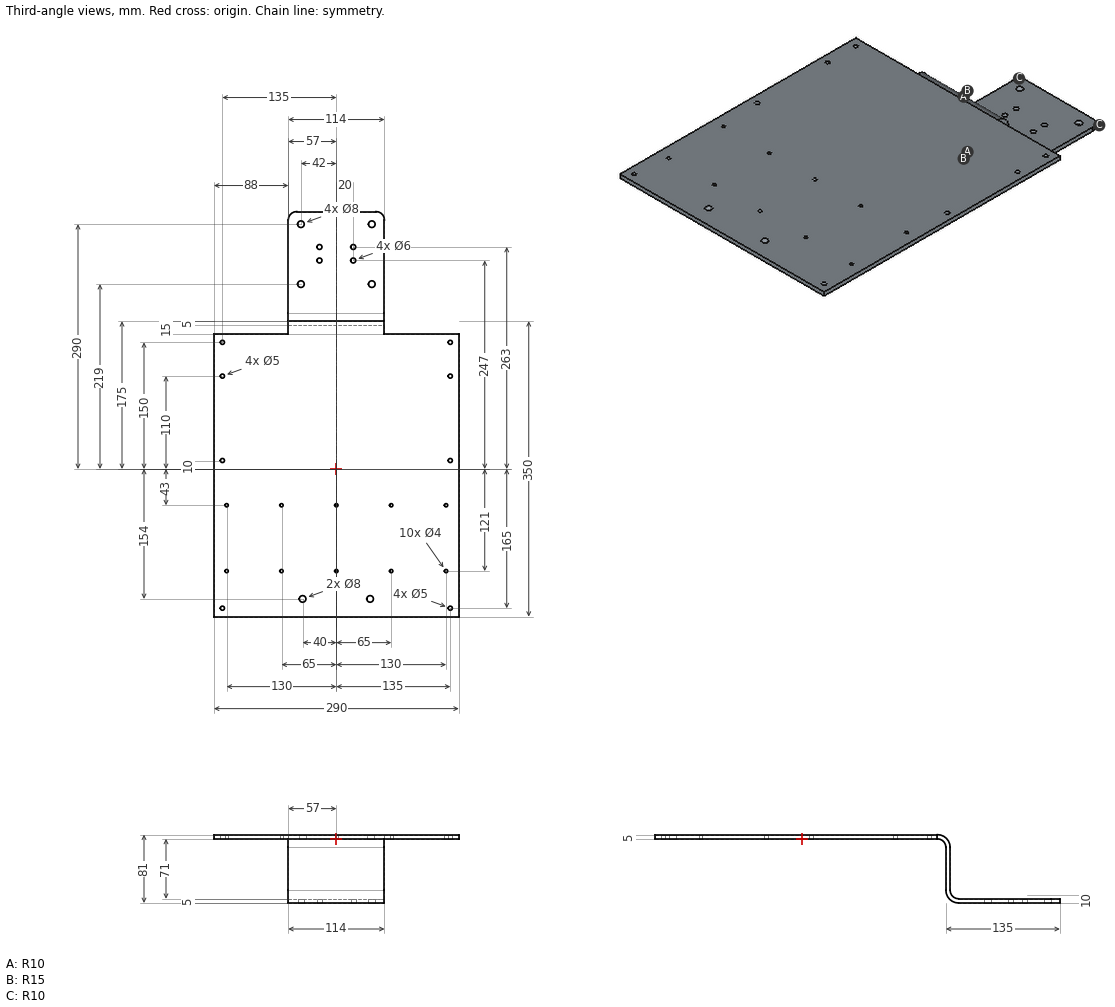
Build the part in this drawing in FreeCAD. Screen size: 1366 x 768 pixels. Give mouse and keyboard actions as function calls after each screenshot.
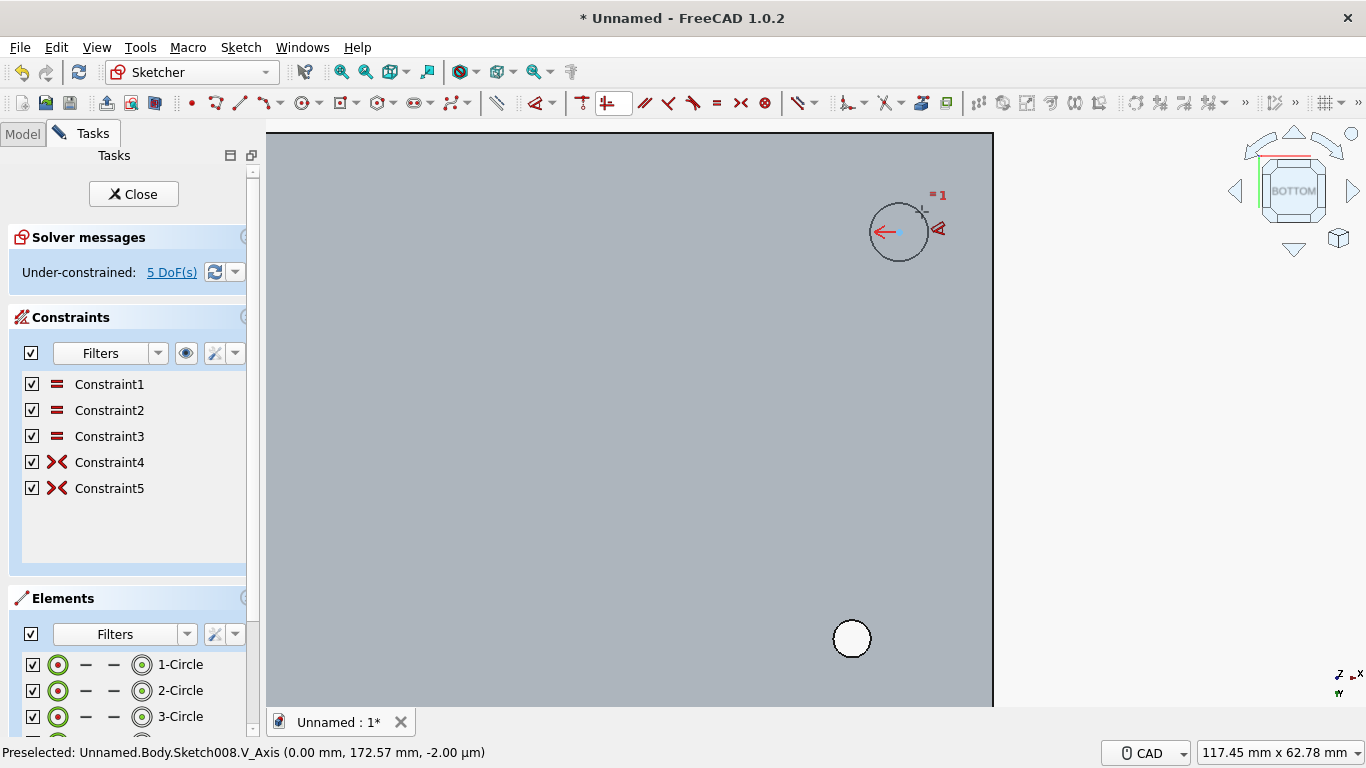
click(920, 212)
click(943, 190)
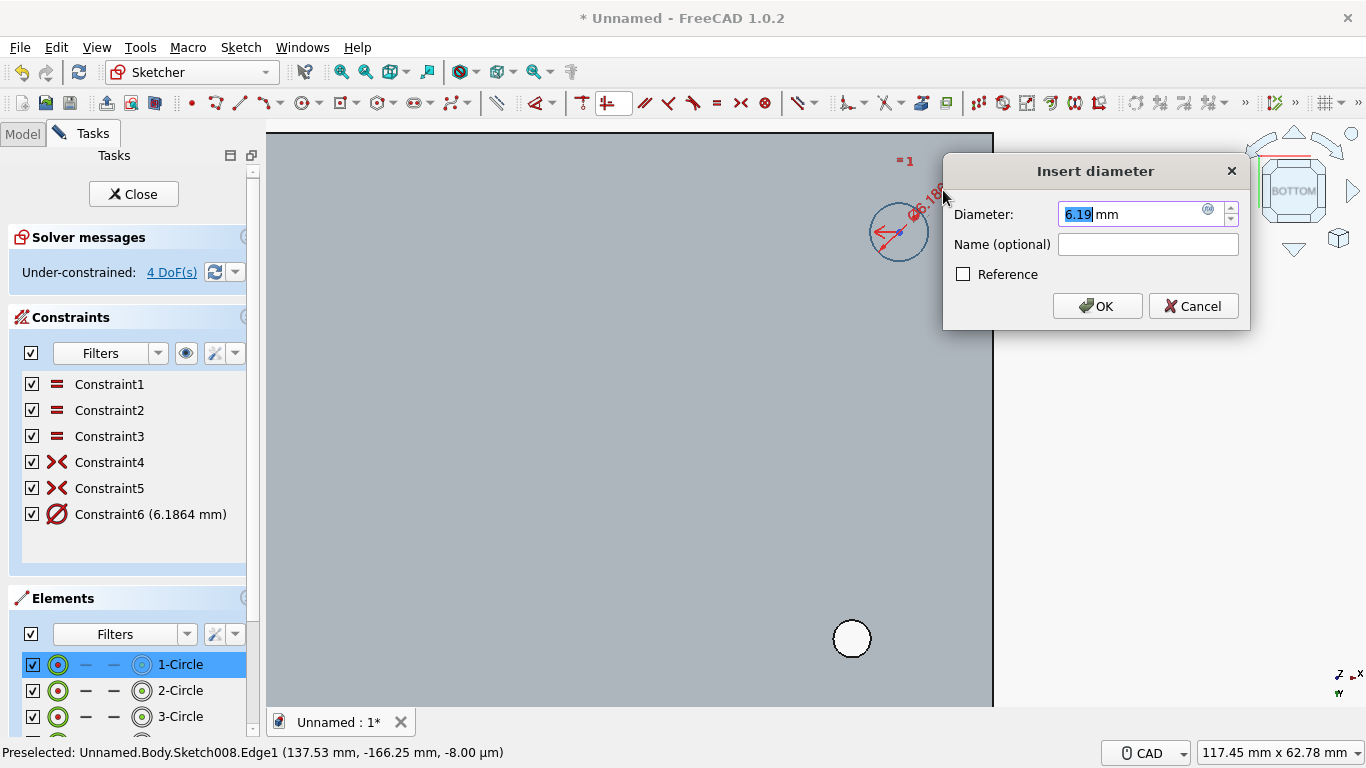
text(5)
key(Return)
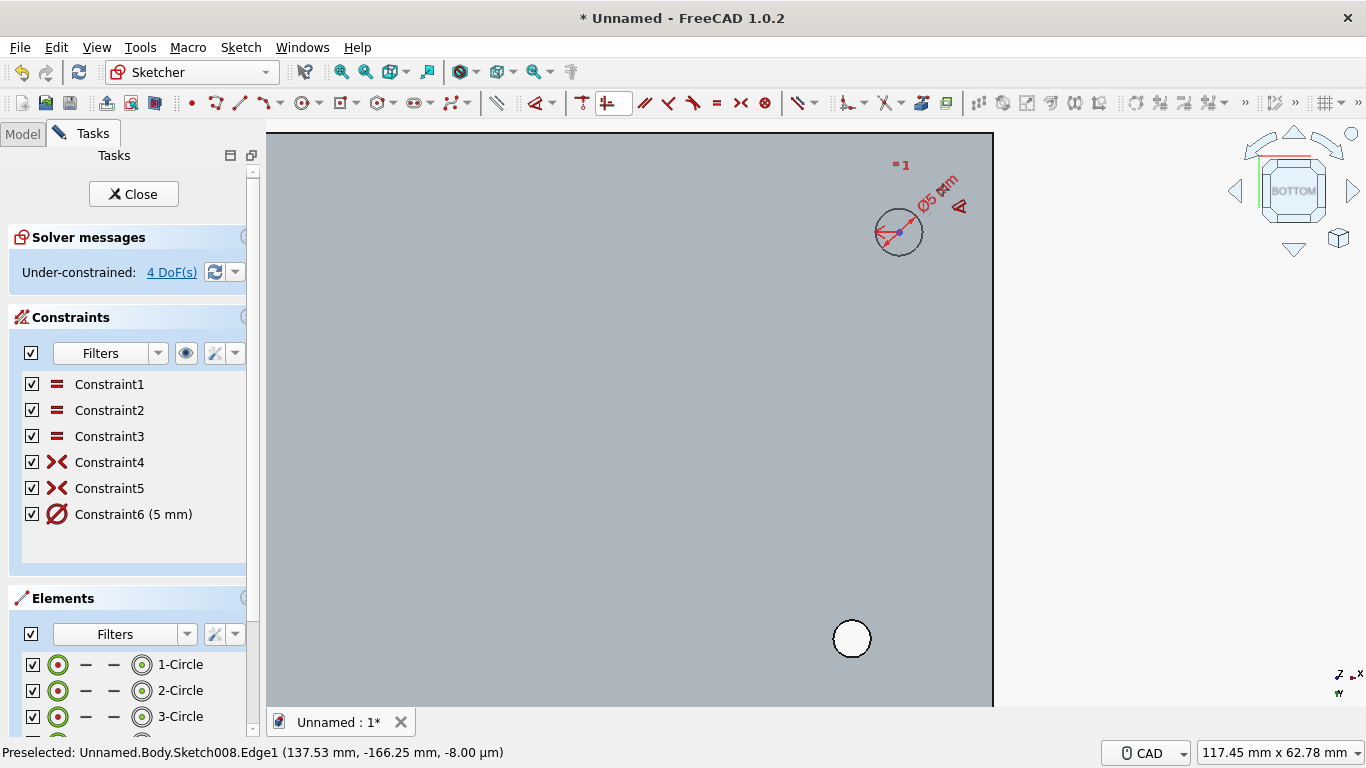
scroll(922, 211, down, 10)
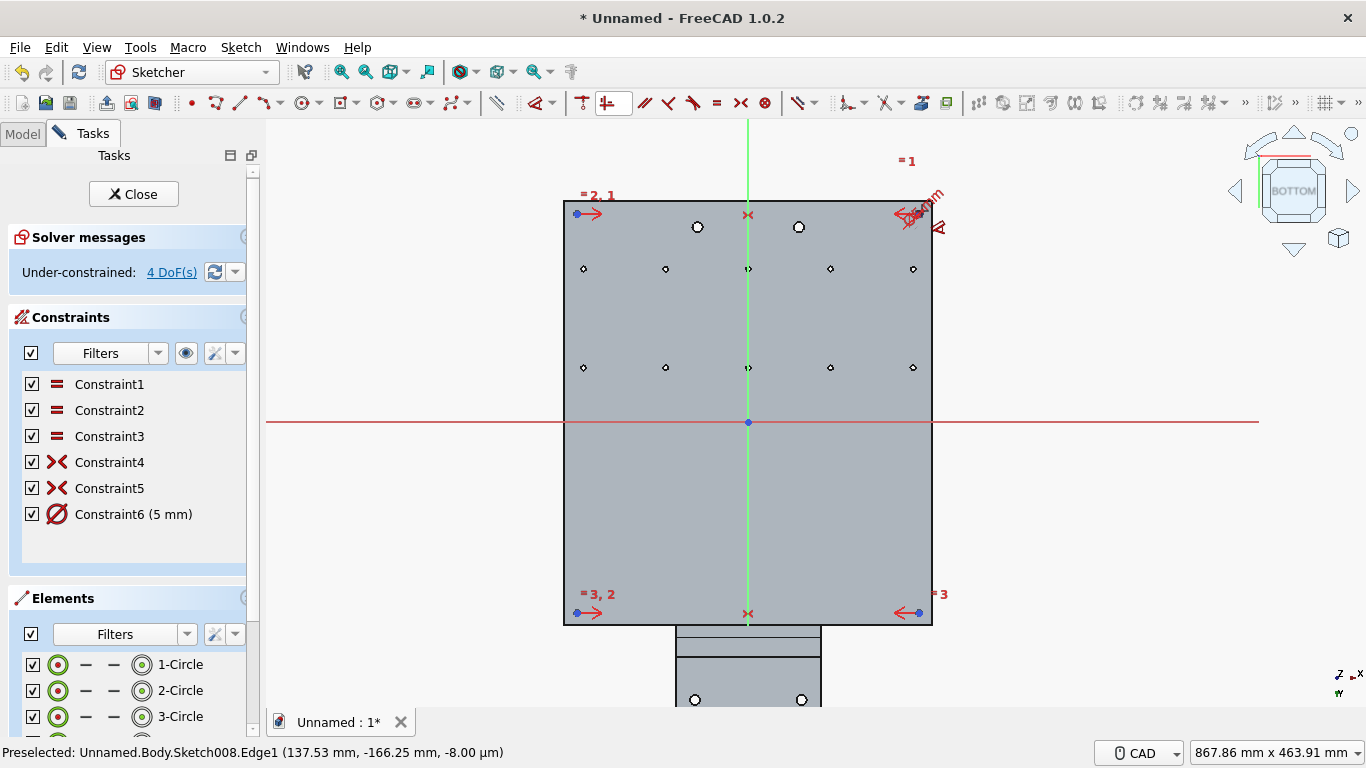
click(919, 214)
click(834, 180)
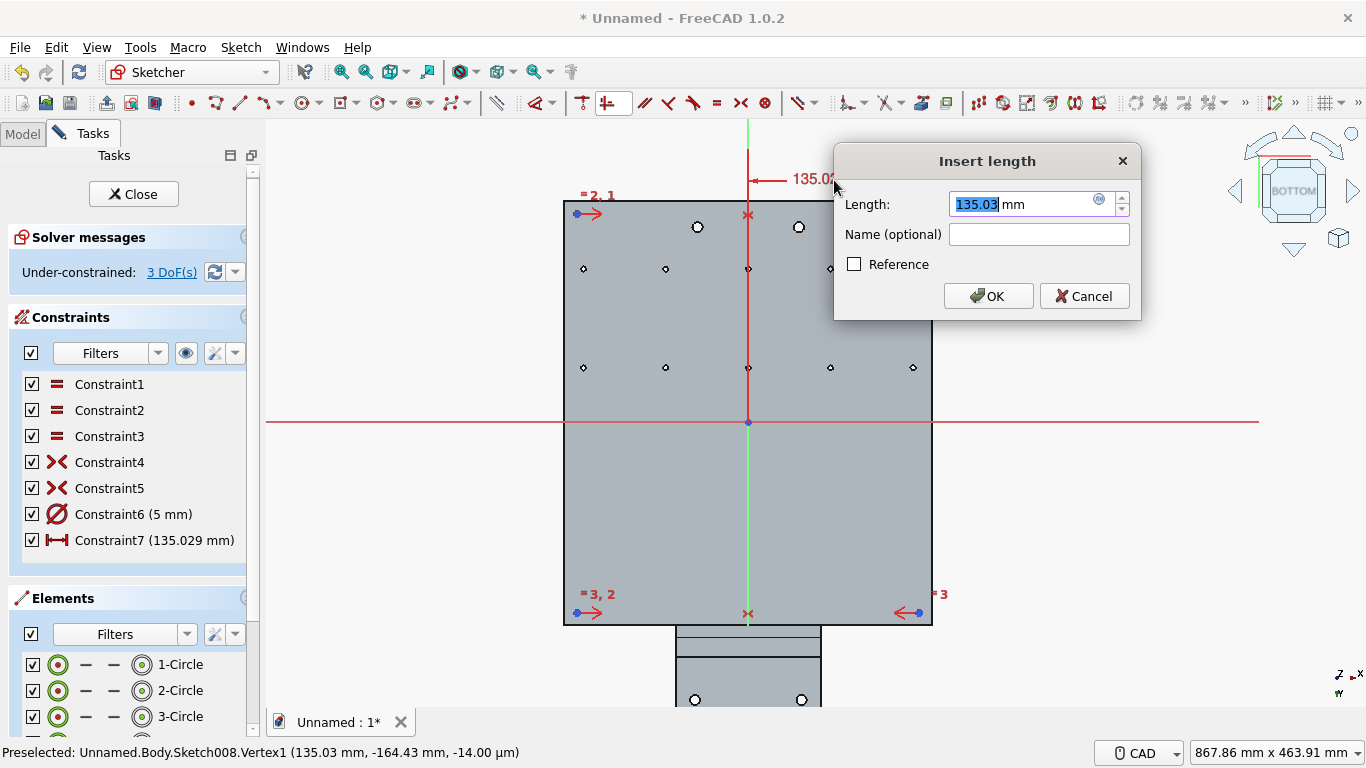
text(135)
key(Return)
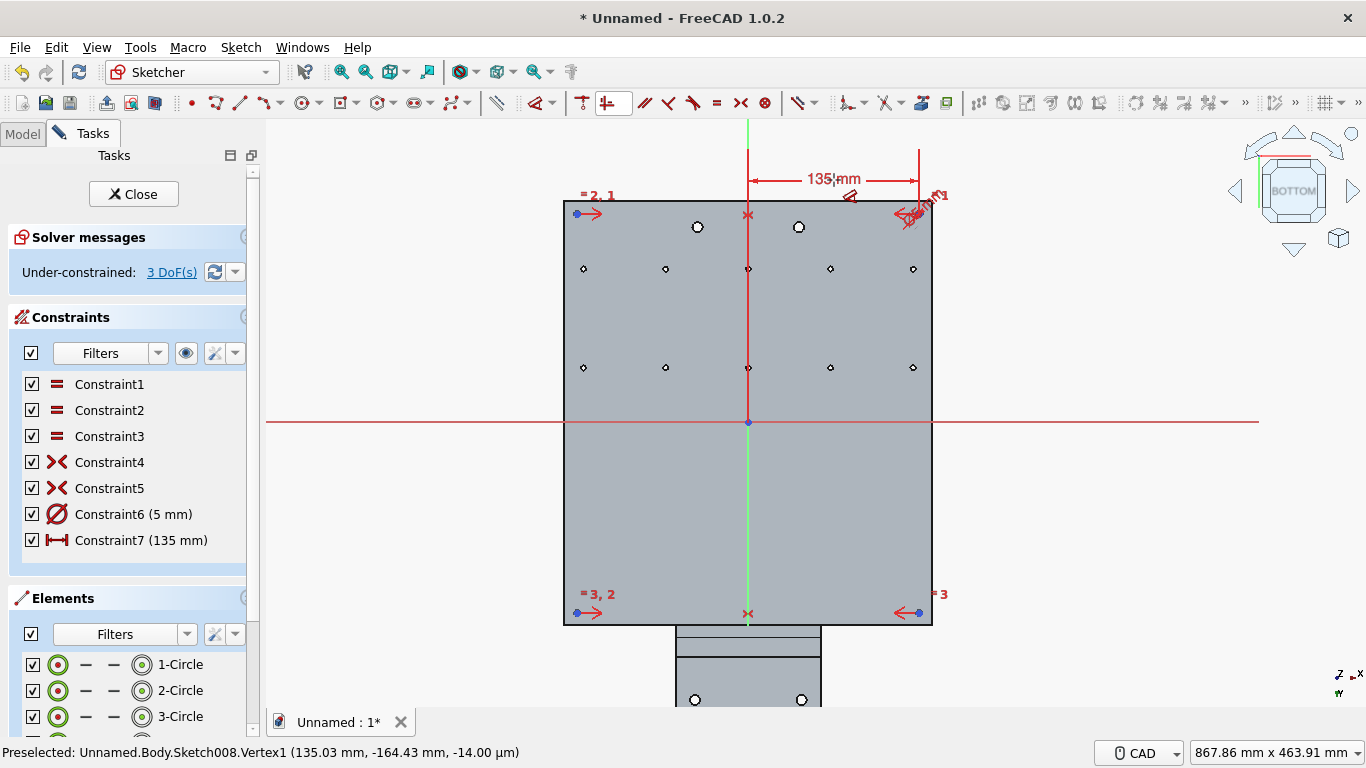
click(919, 214)
click(953, 318)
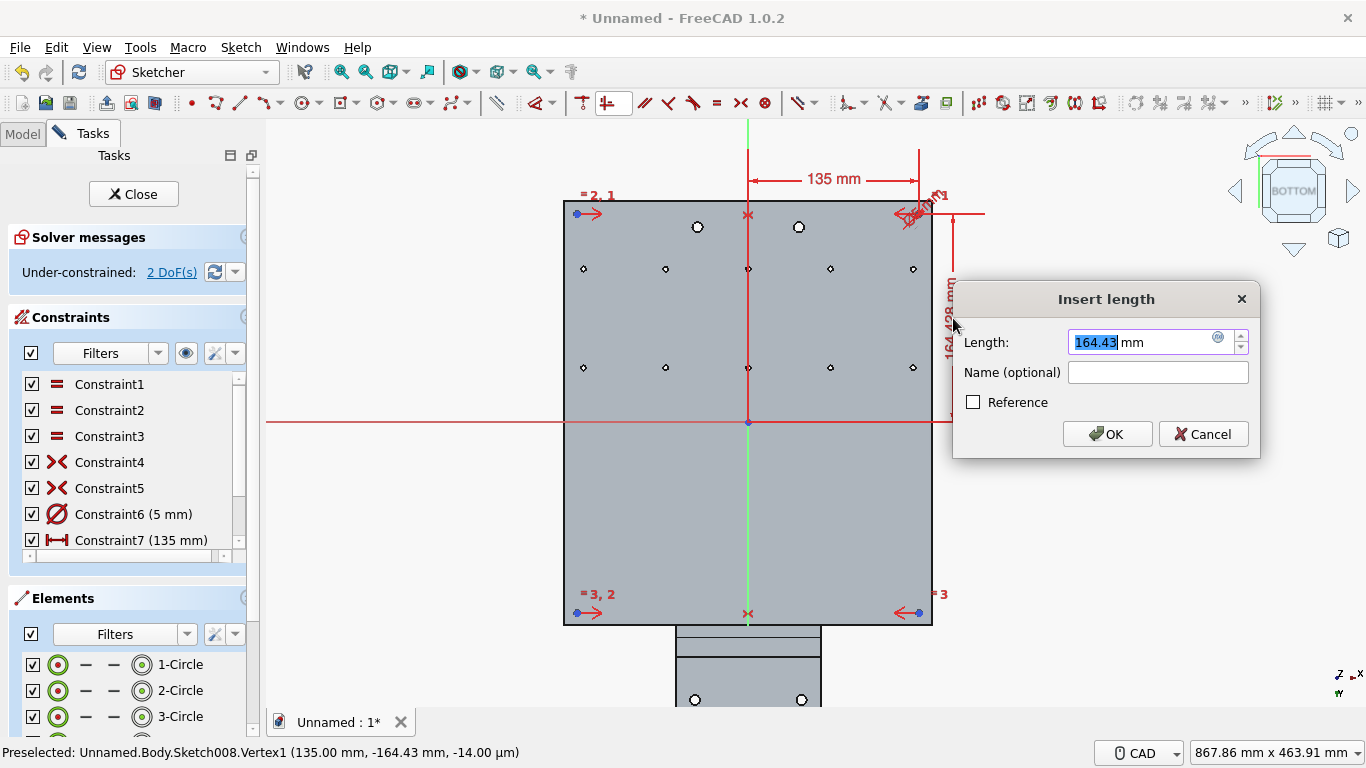
text(165)
key(Return)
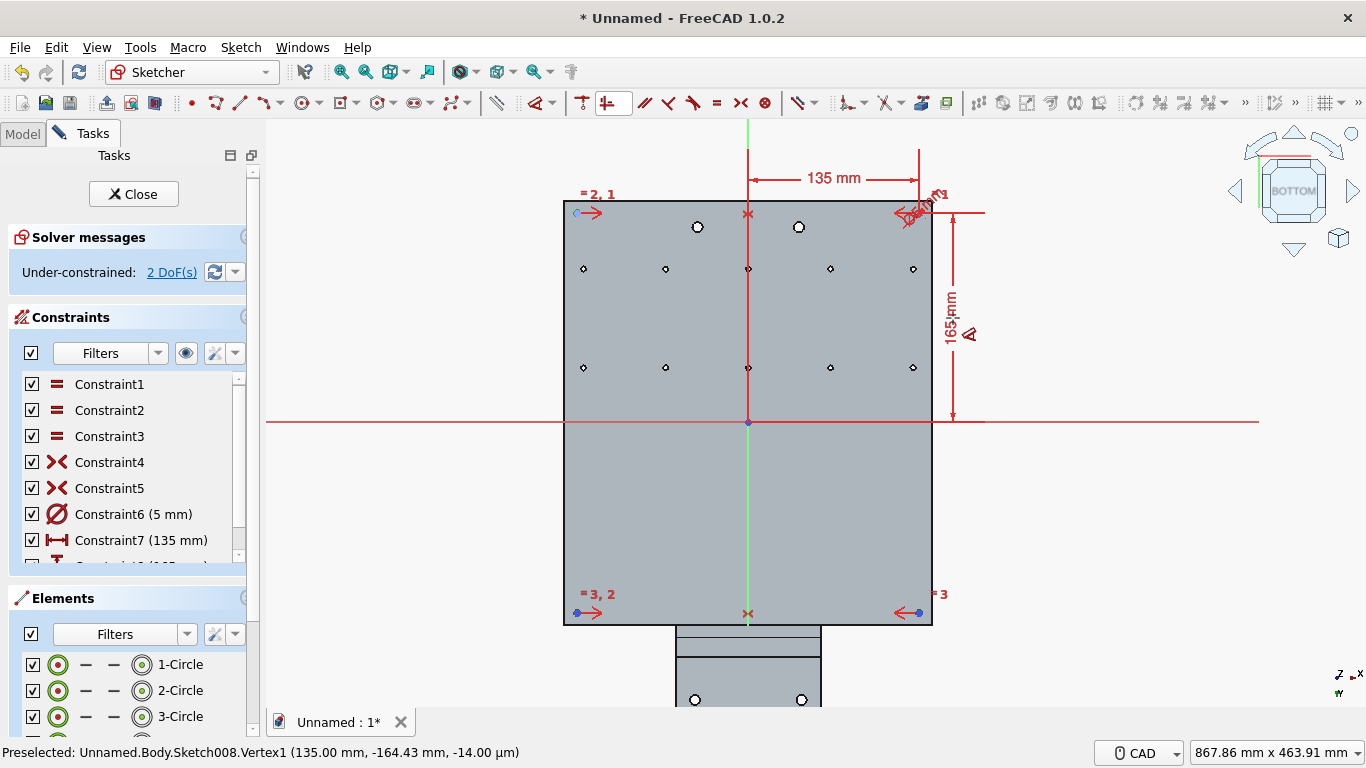
click(577, 613)
click(663, 647)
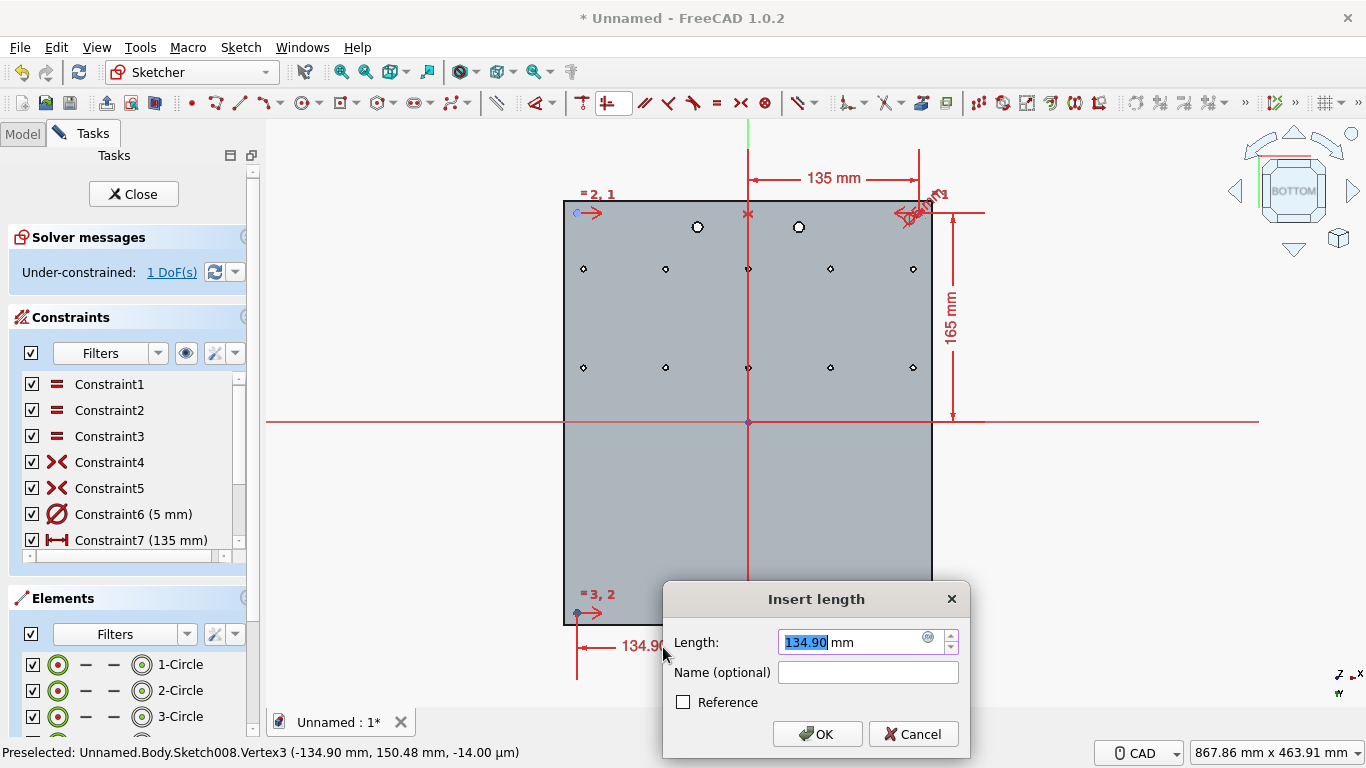
text(135)
key(Return)